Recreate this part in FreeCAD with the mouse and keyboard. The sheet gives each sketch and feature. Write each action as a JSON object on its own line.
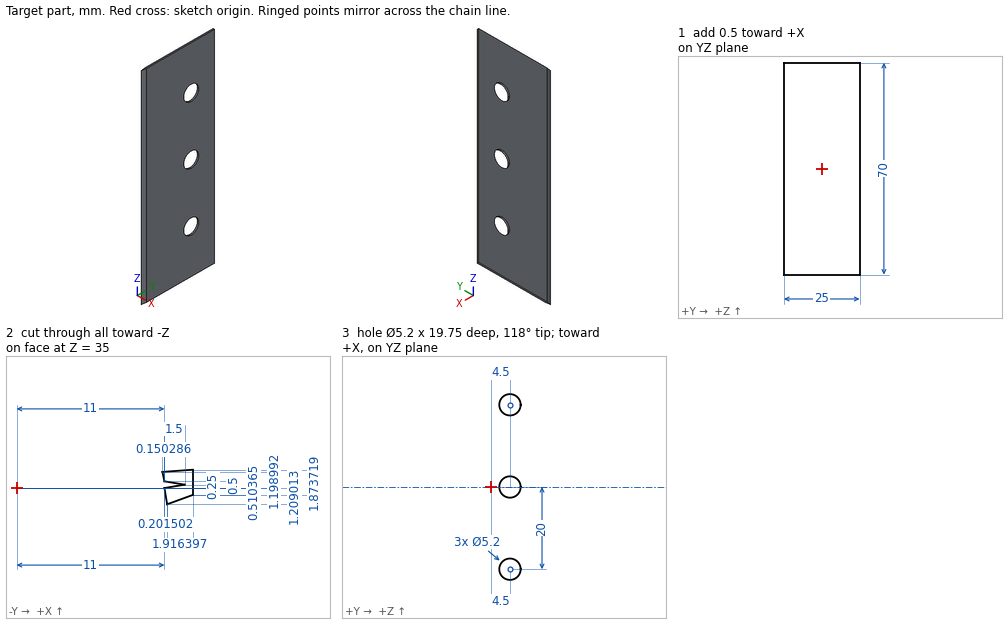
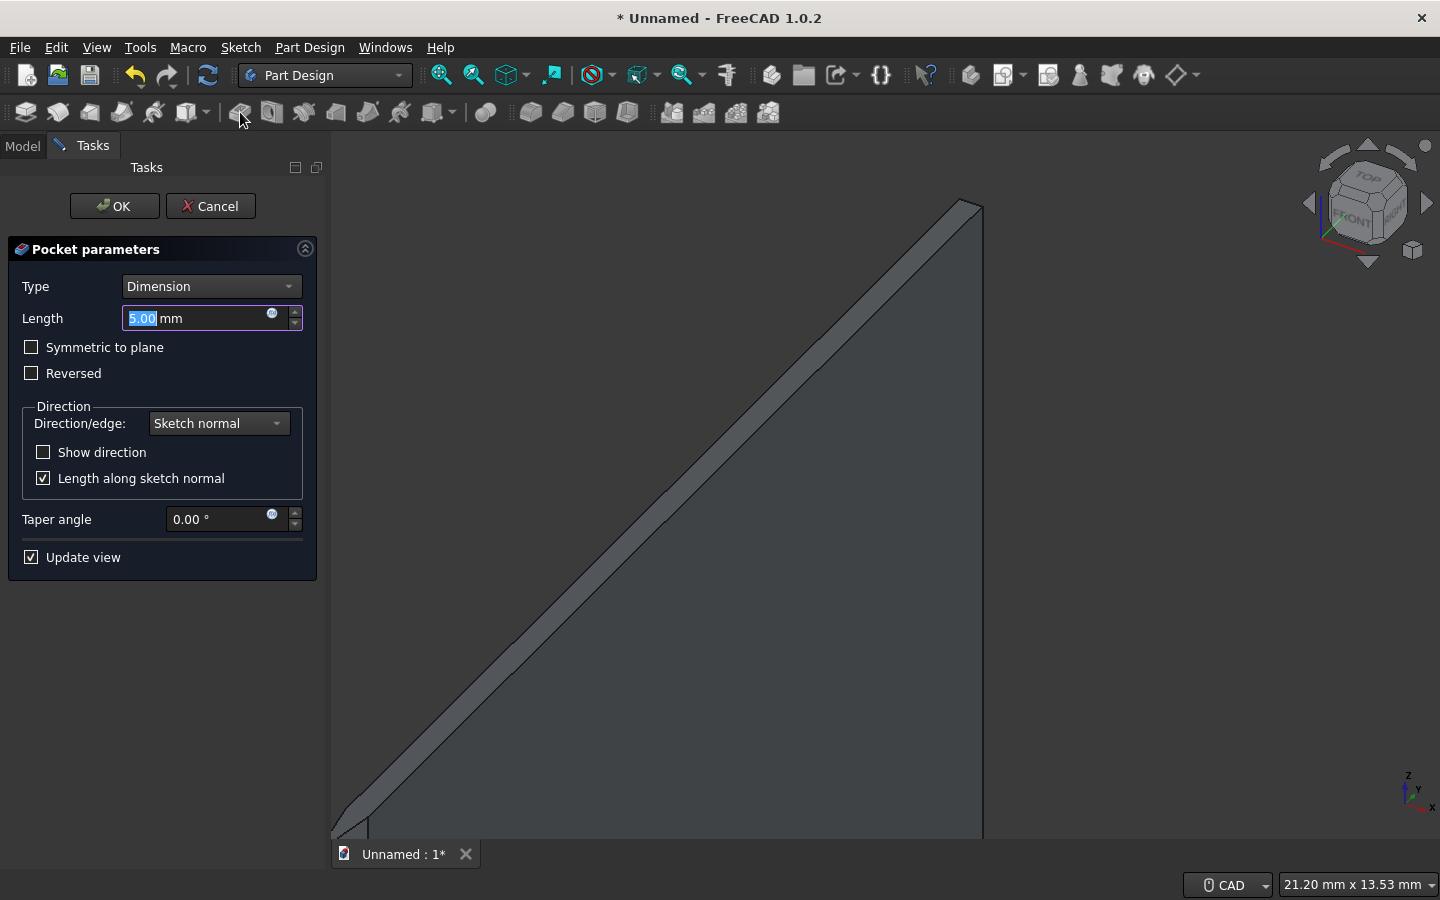
{"action": "left_click", "coordinate": [212, 286]}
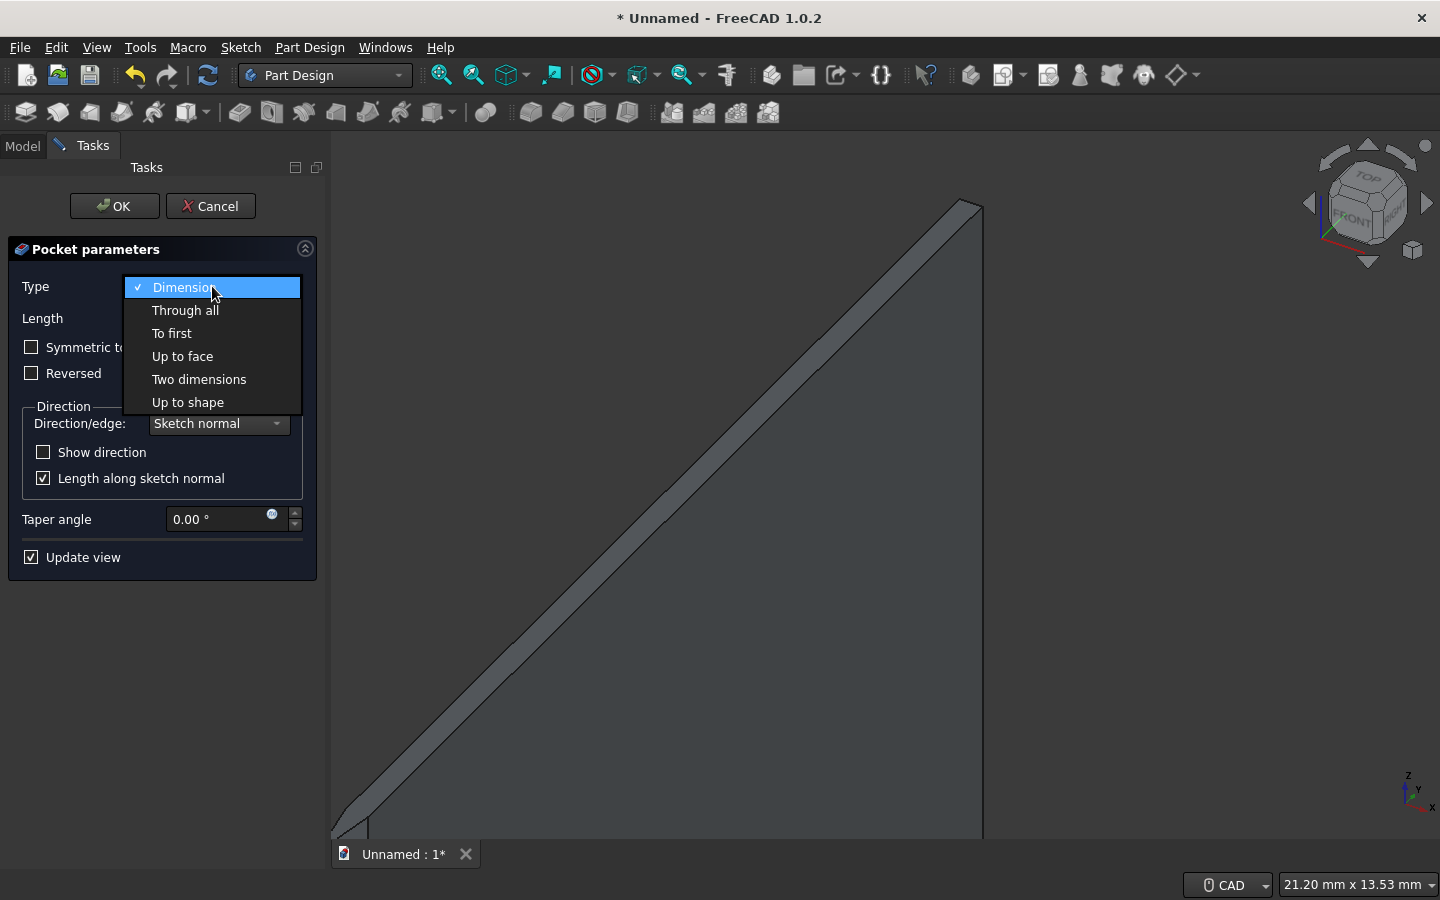
{"action": "left_click", "coordinate": [212, 310]}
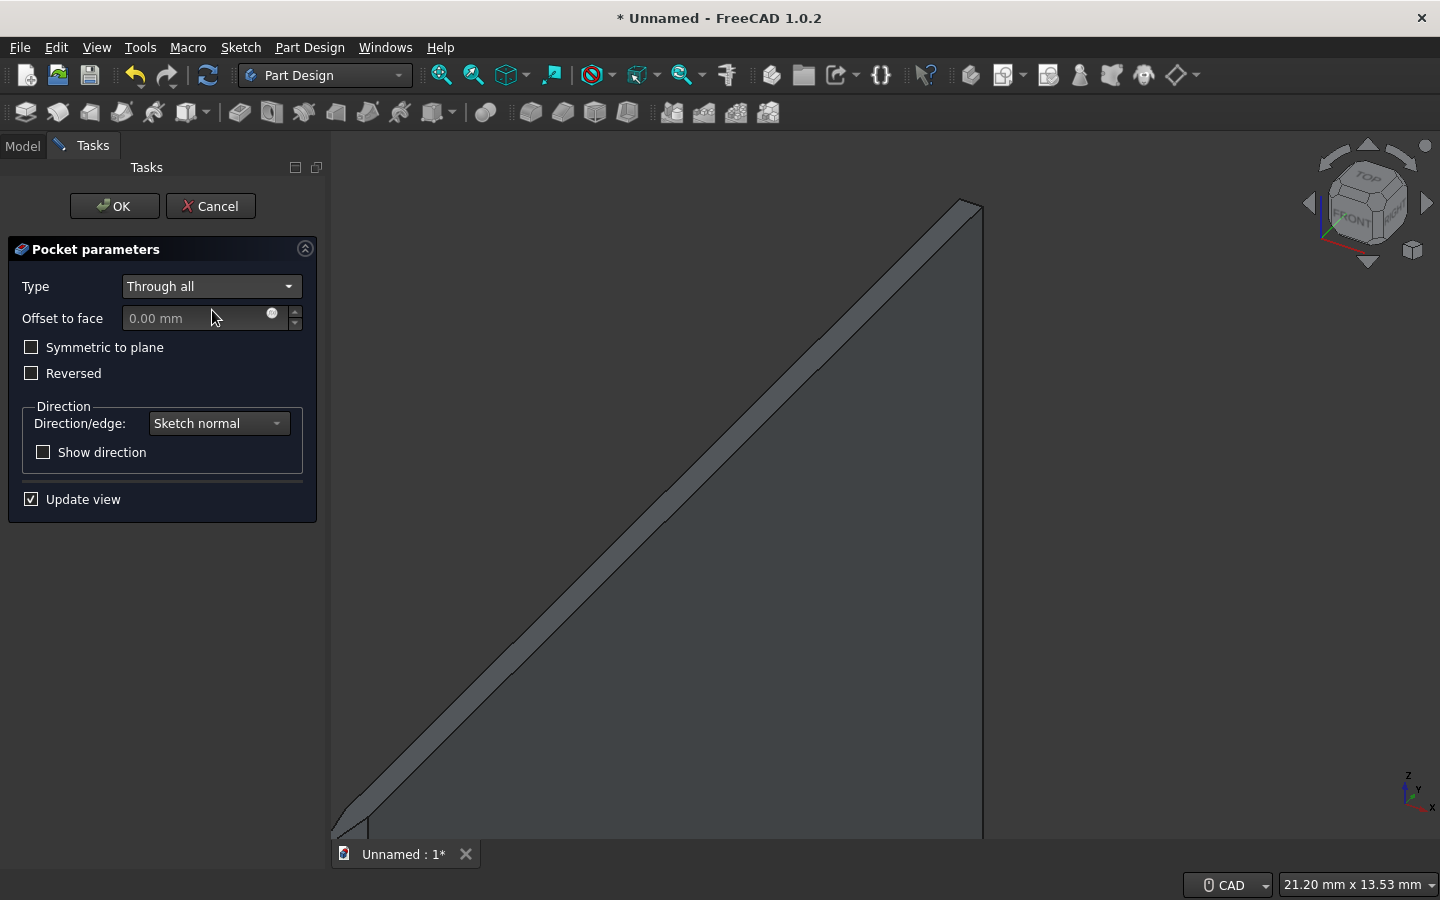
{"action": "left_click", "coordinate": [115, 206]}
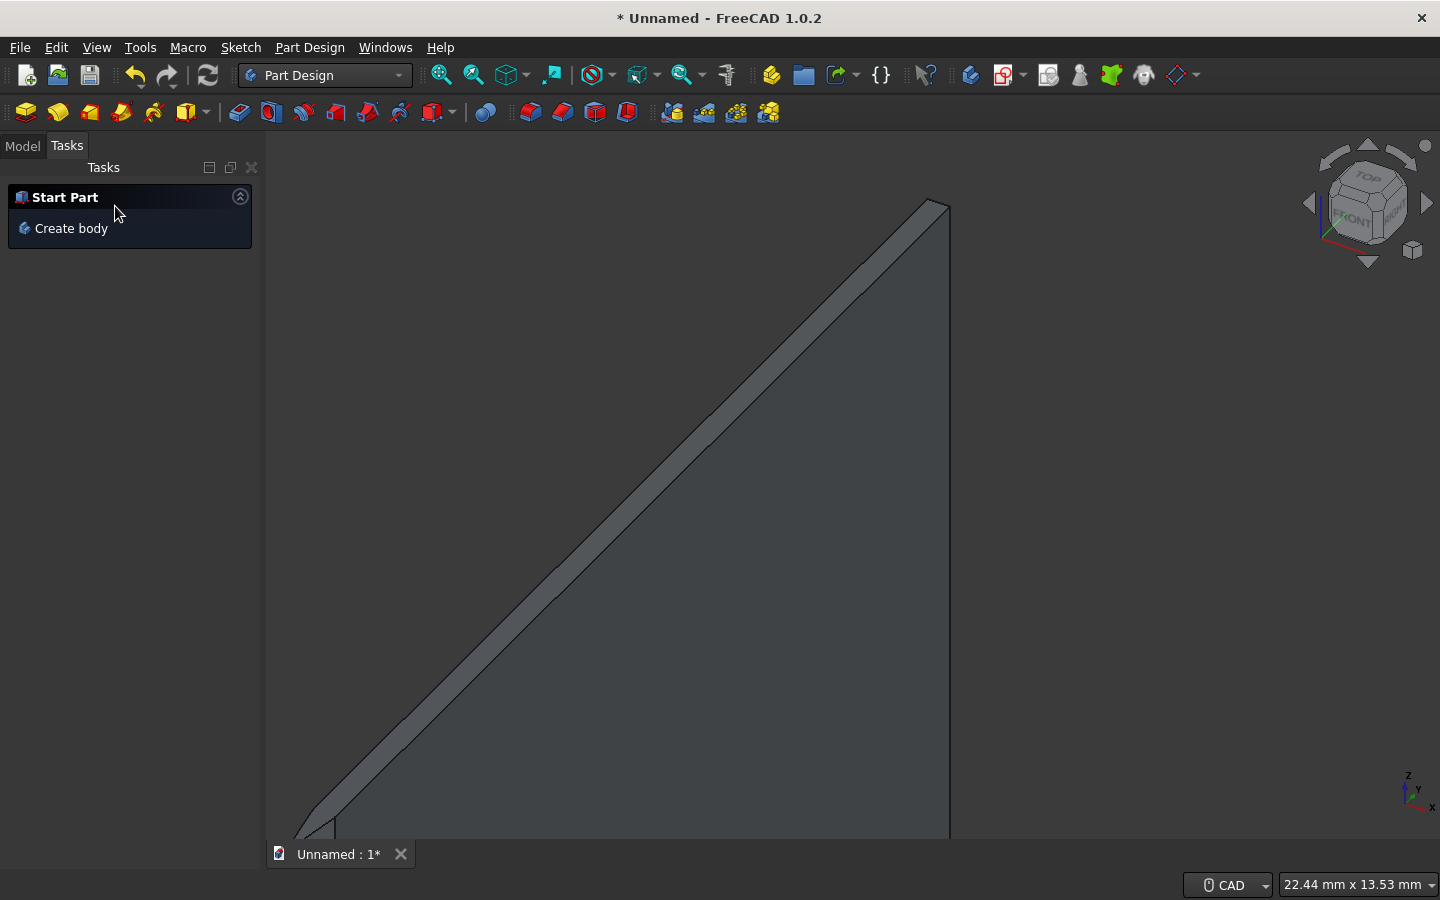
{"action": "left_click", "coordinate": [442, 76]}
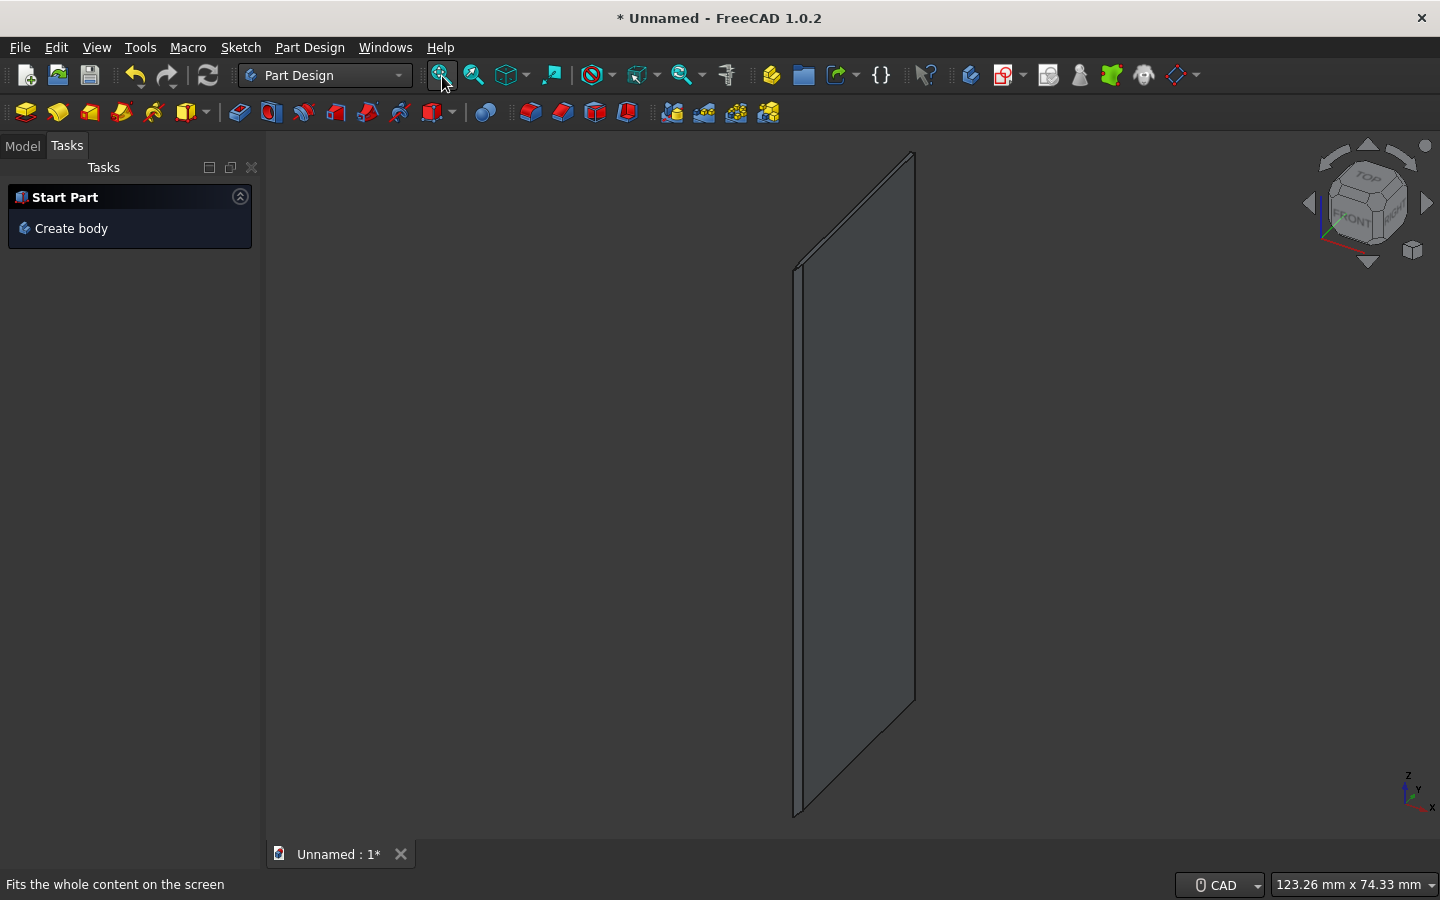
{"action": "left_click", "coordinate": [1004, 76]}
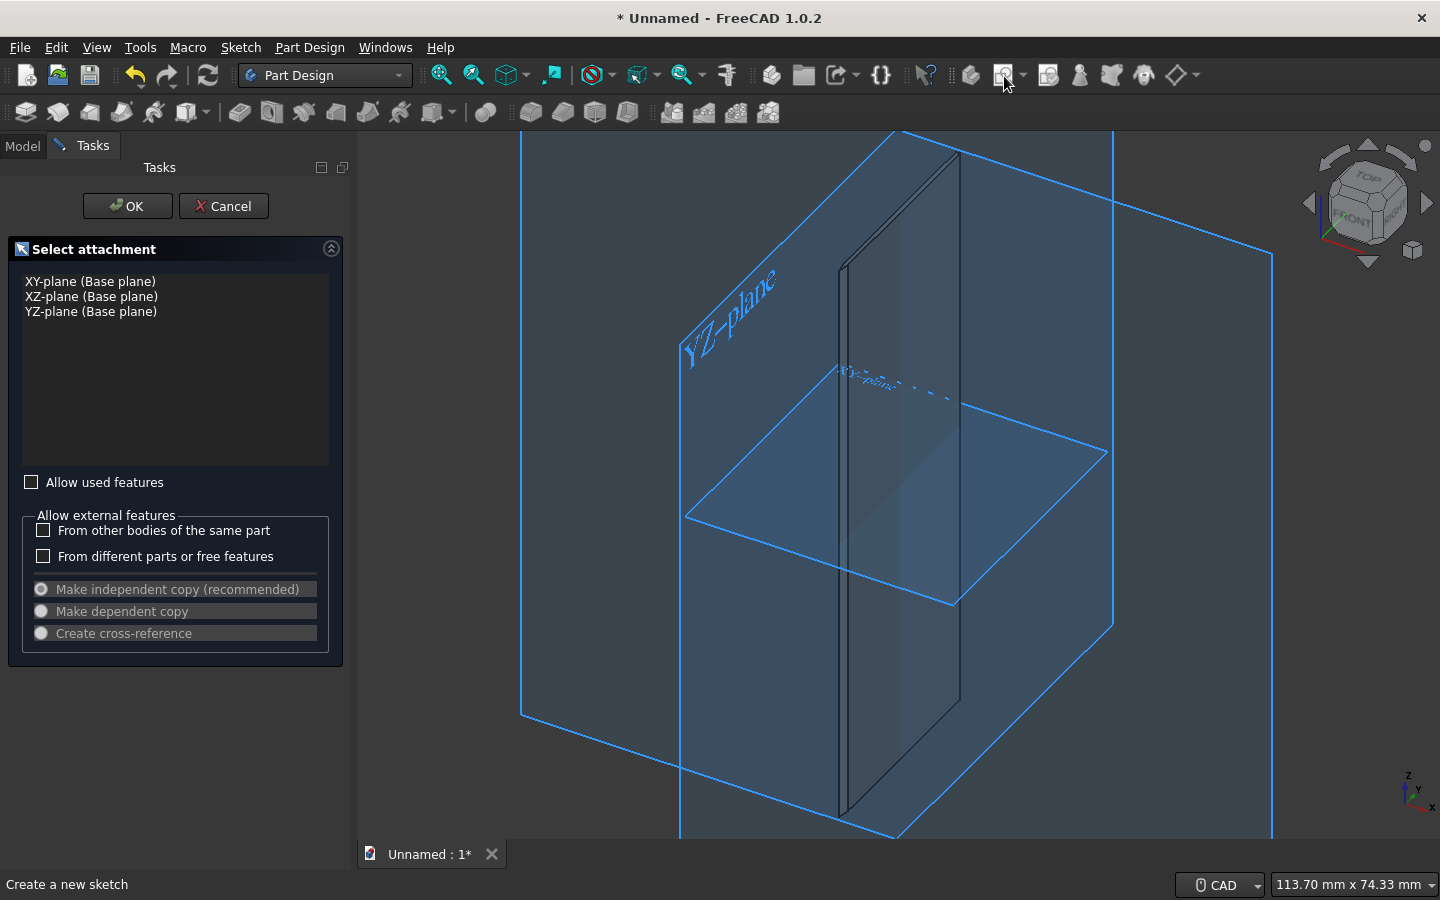
{"action": "left_click", "coordinate": [82, 312]}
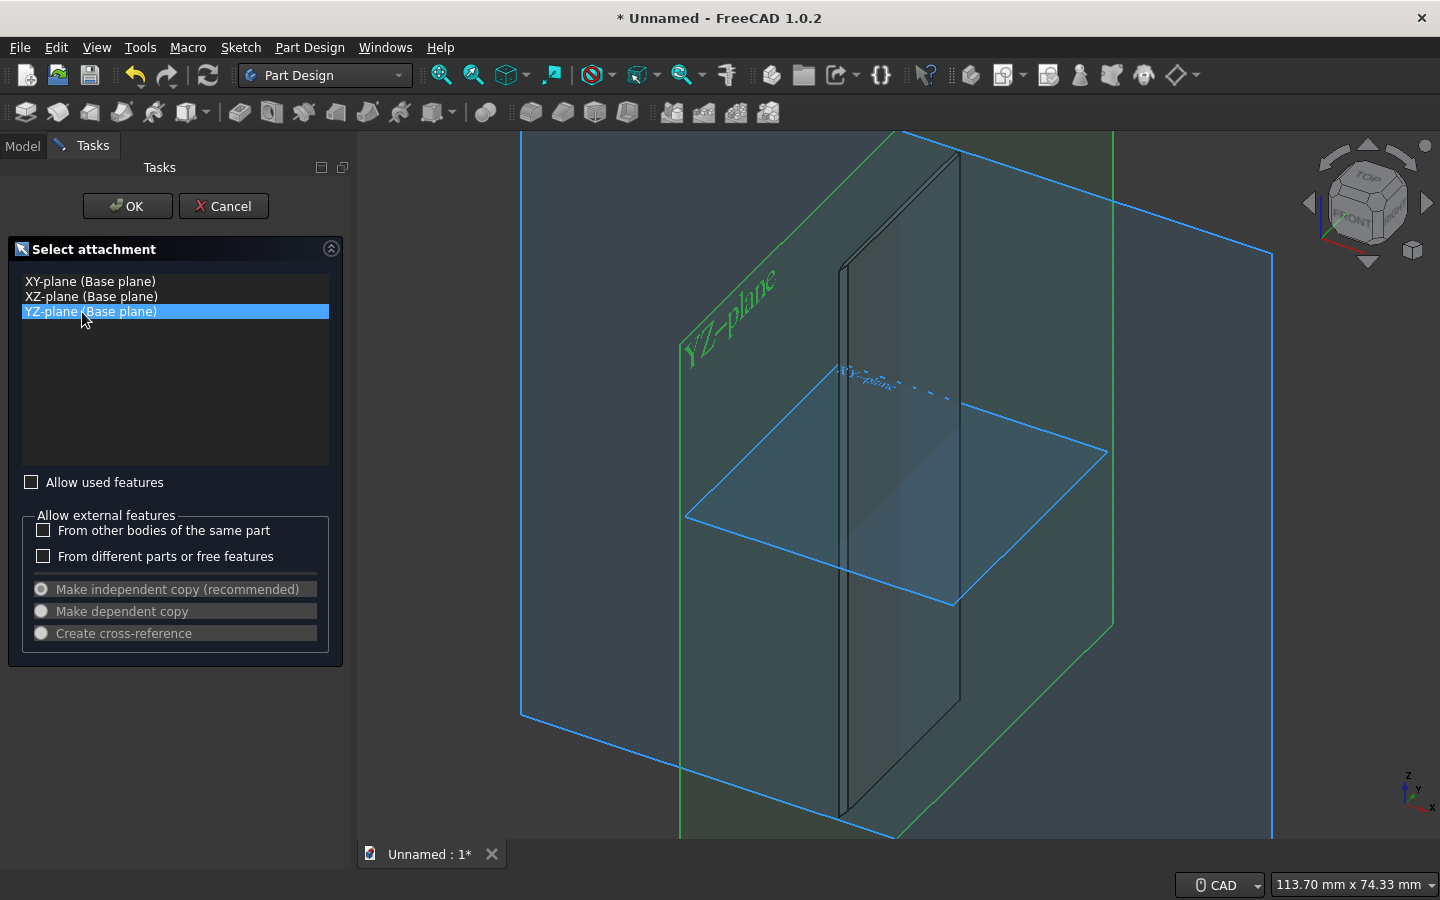
{"action": "left_click", "coordinate": [128, 206]}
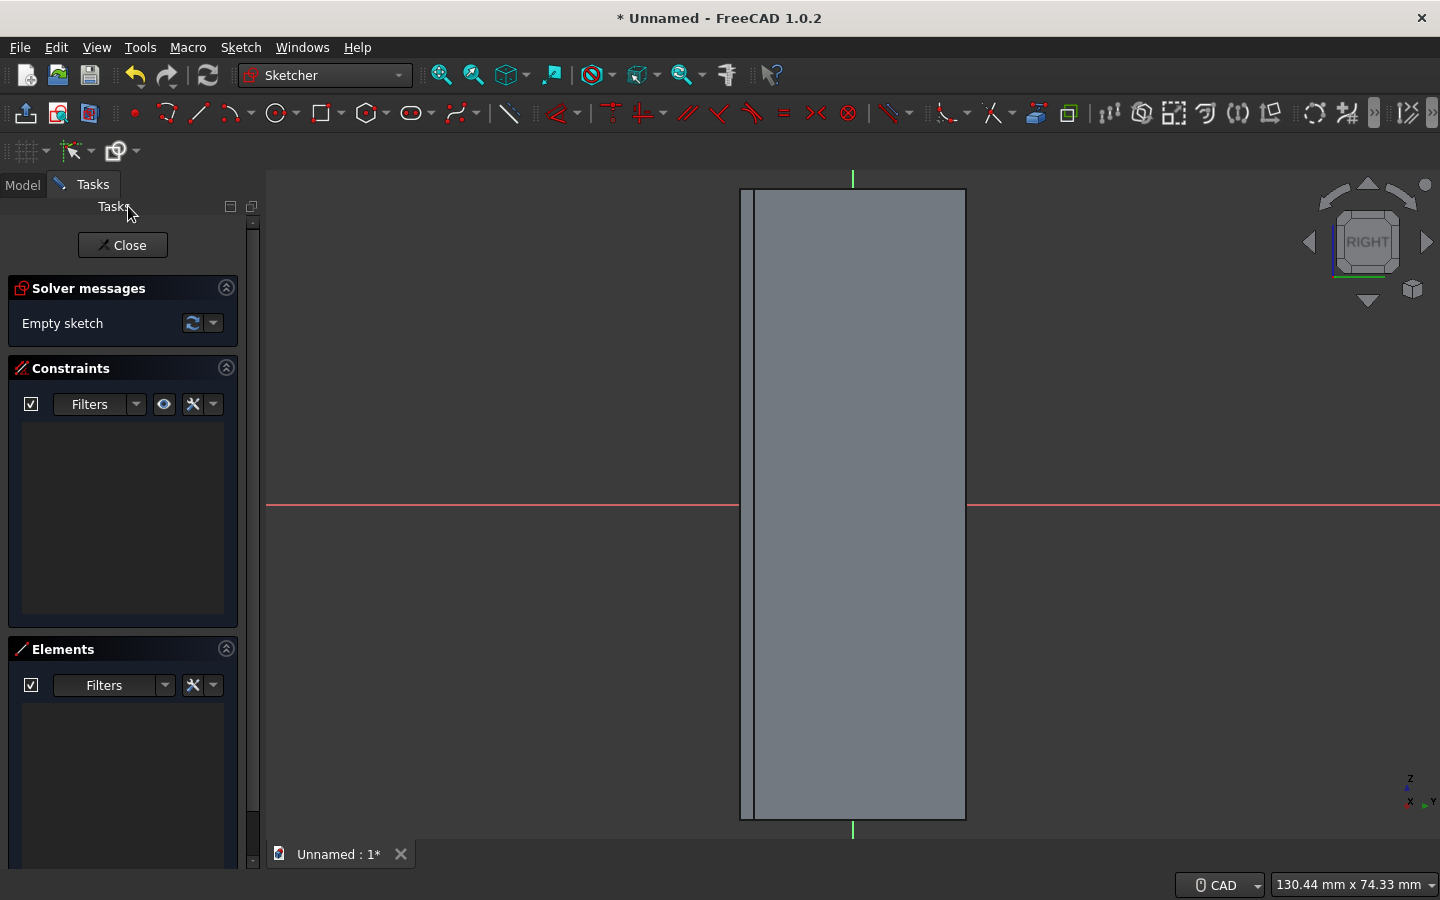
{"action": "key", "text": "q s"}